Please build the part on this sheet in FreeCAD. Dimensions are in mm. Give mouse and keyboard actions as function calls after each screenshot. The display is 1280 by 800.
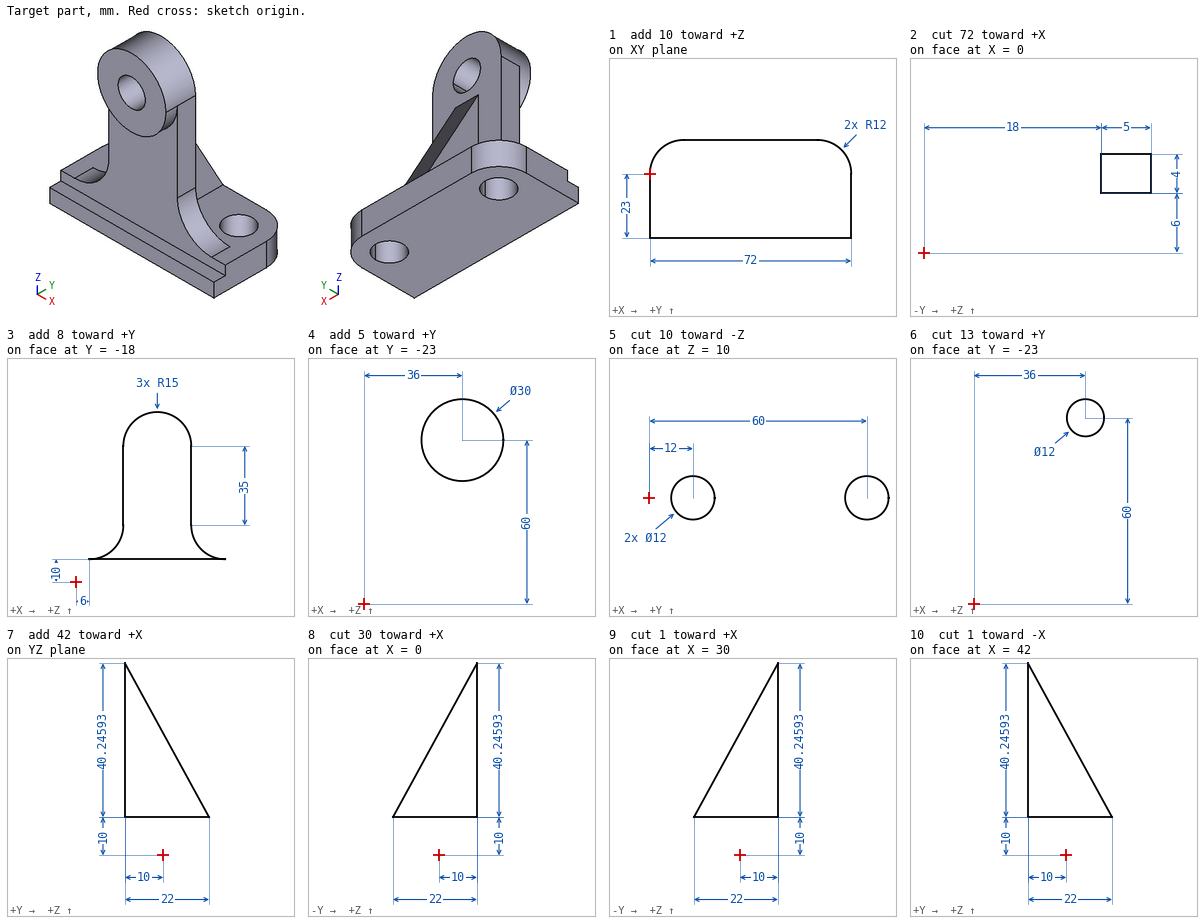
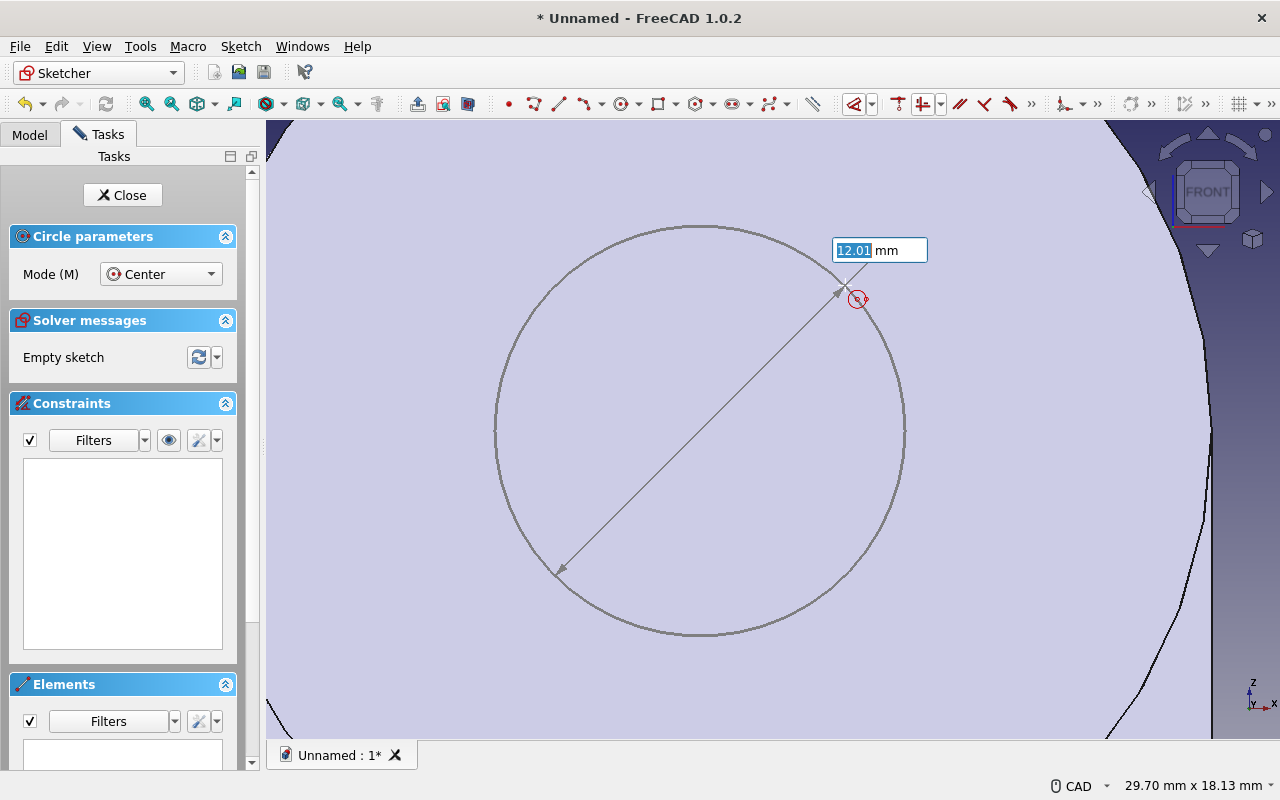
text(12)
key(Return)
key(Escape)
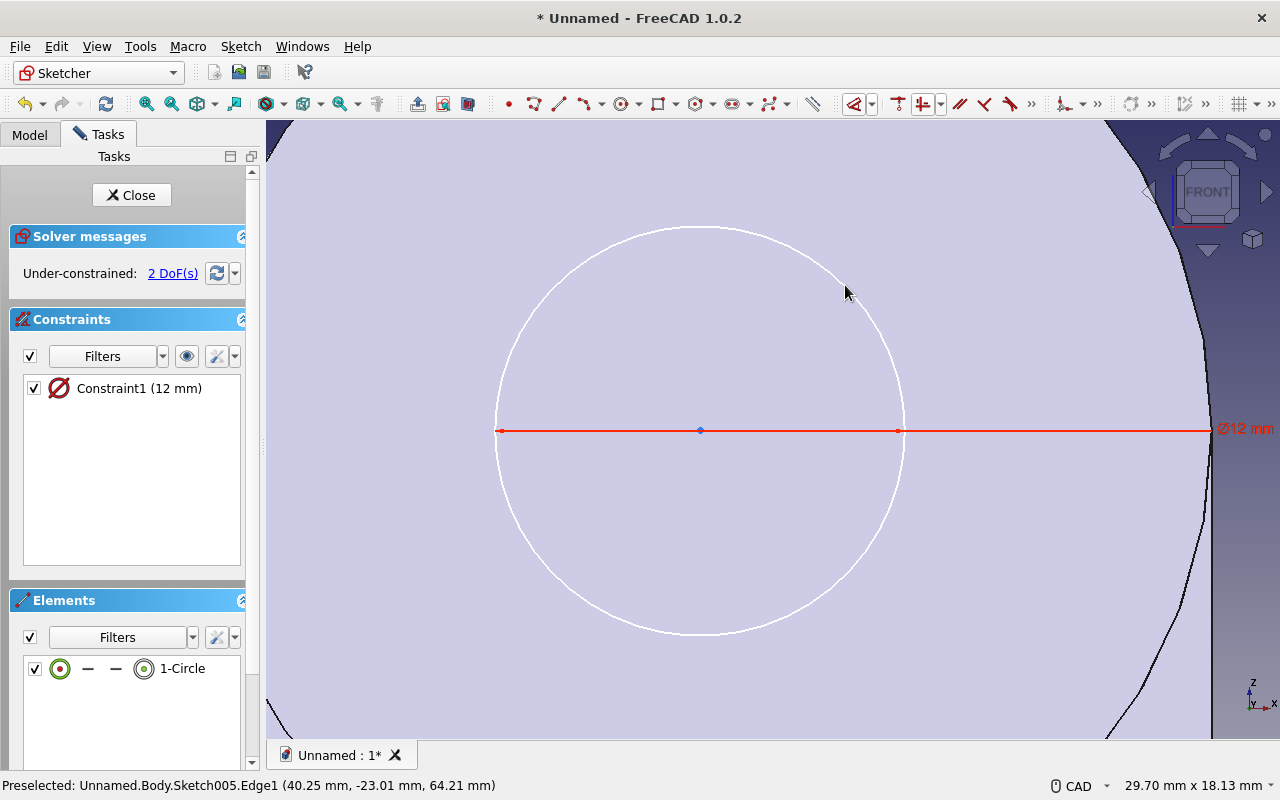
click(700, 431)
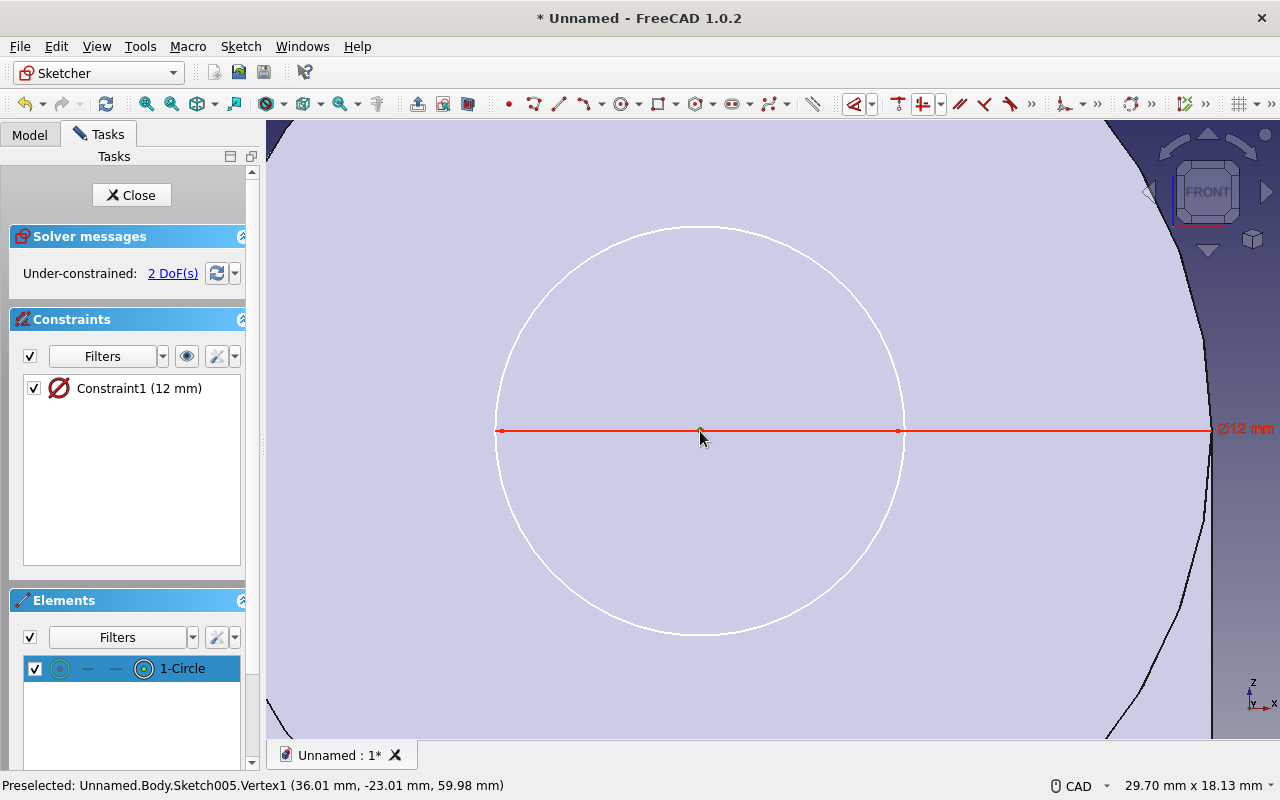
click(872, 104)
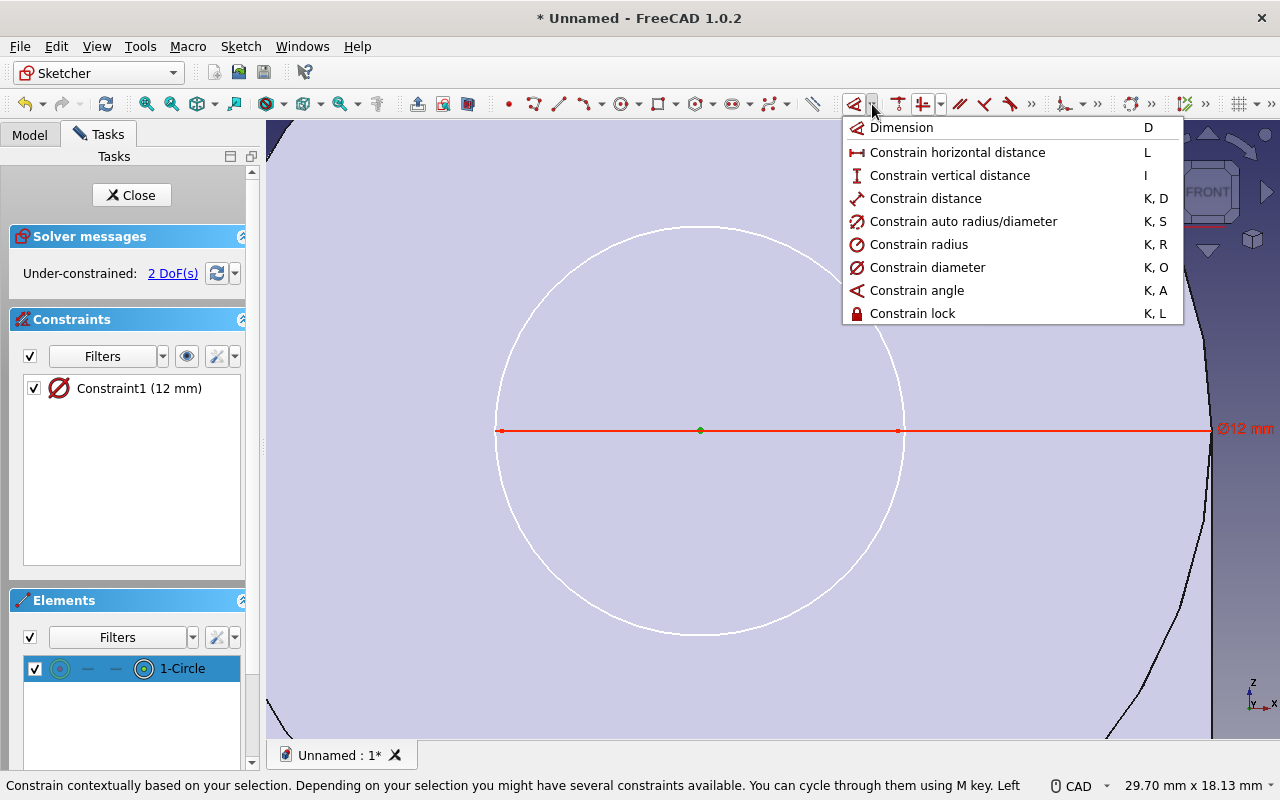
click(1013, 152)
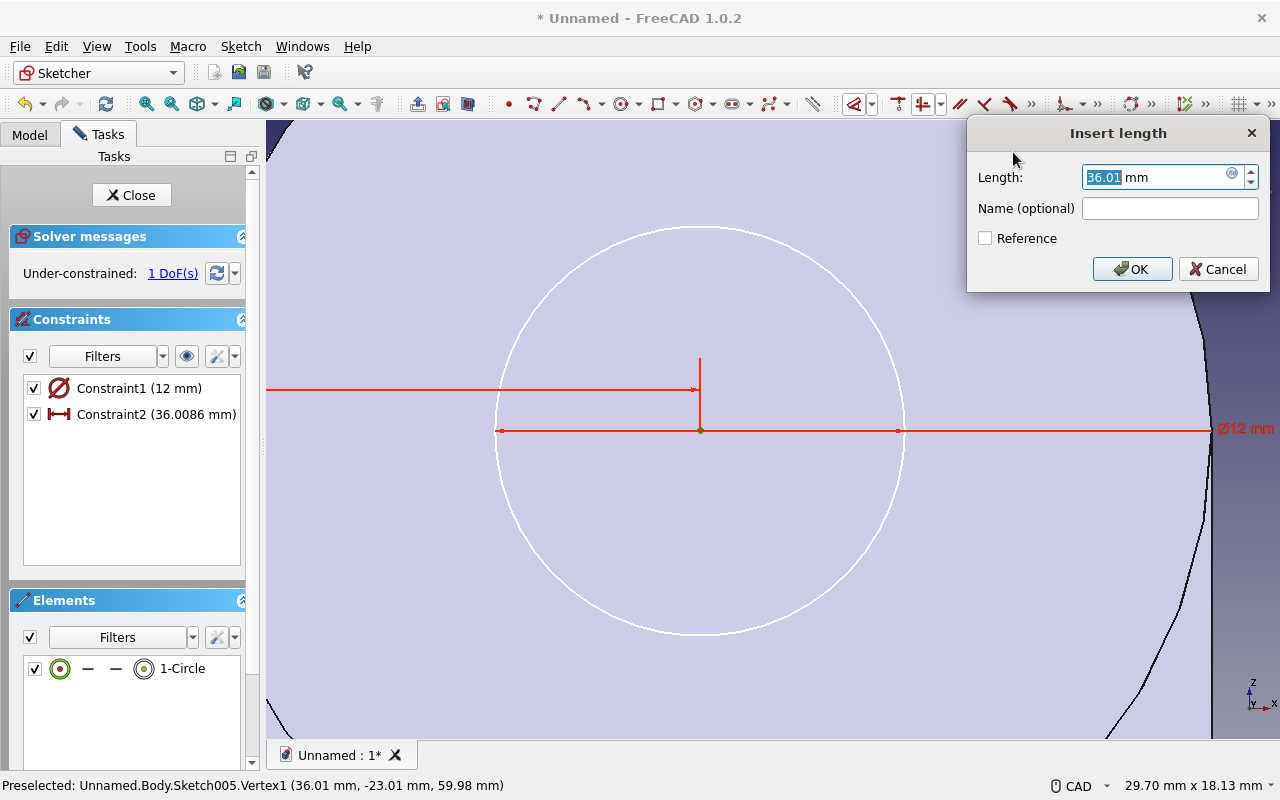
text(36)
key(Return)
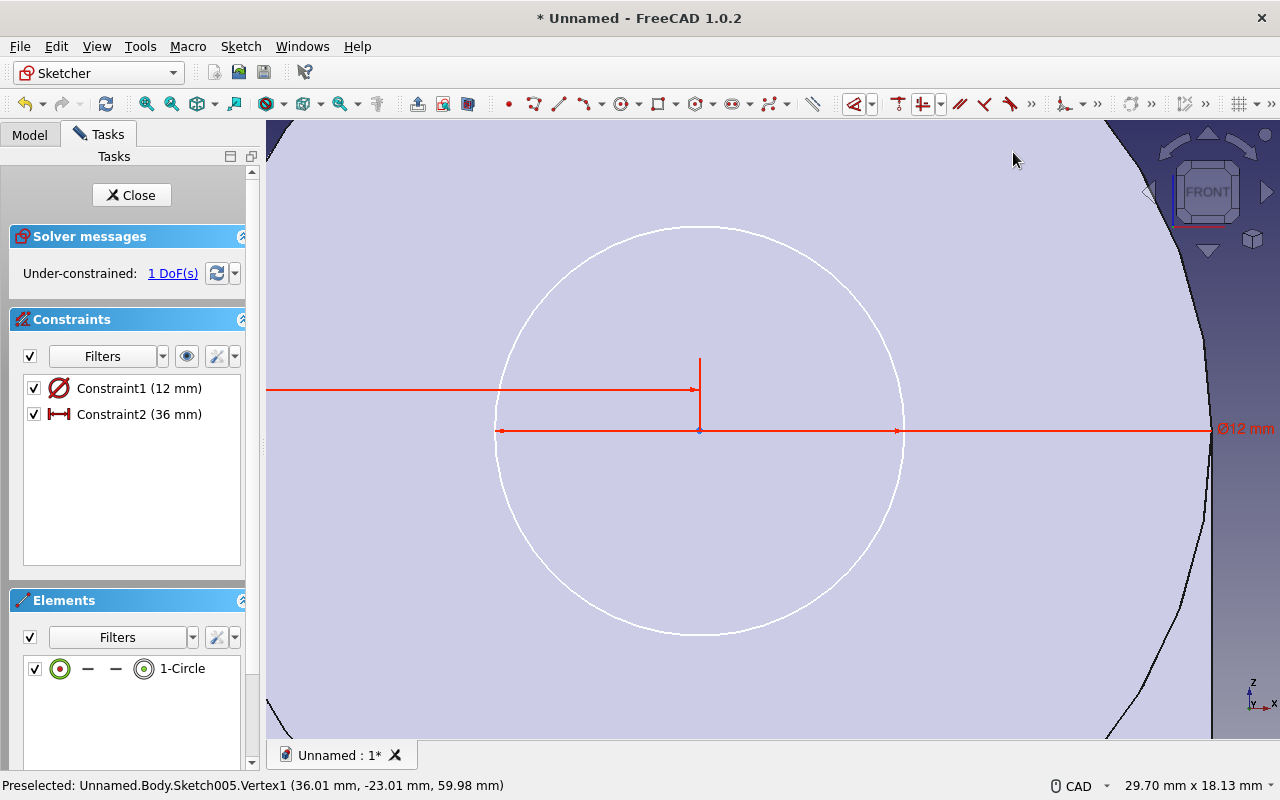
click(700, 431)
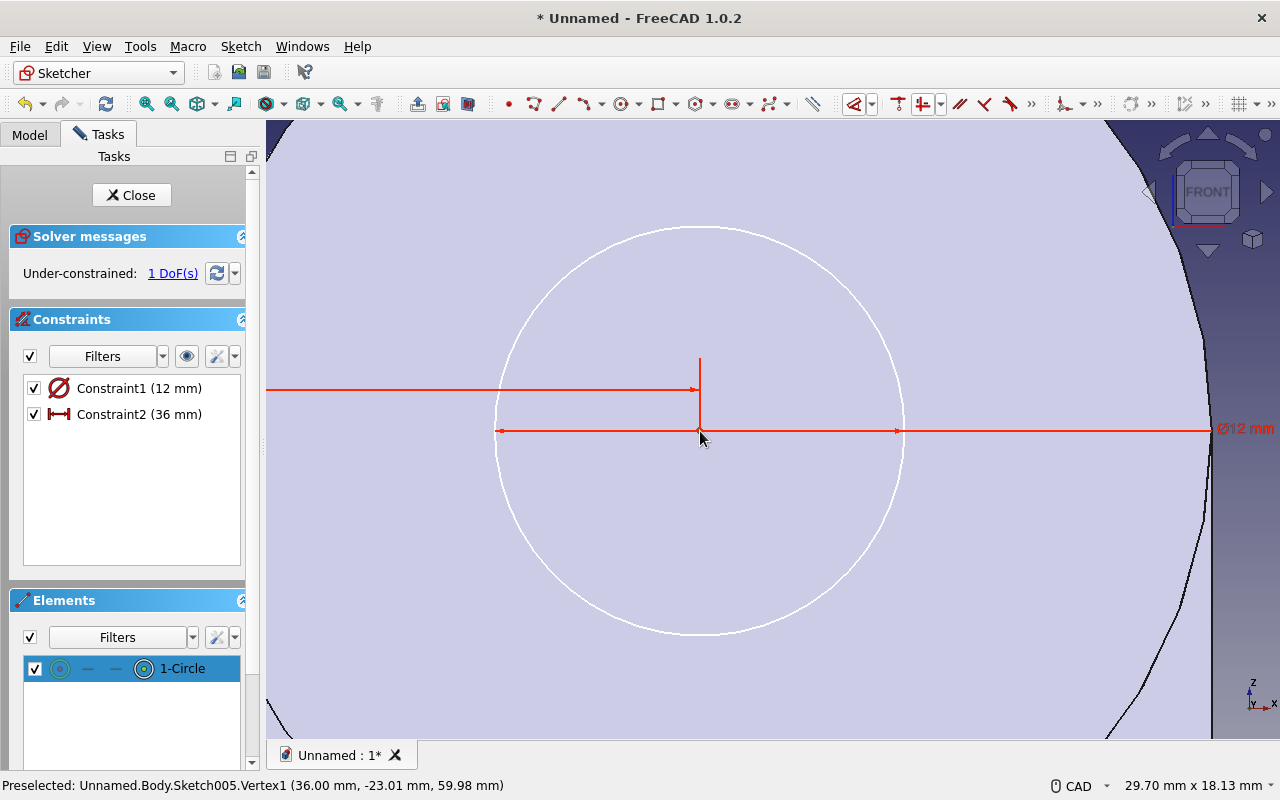
click(872, 104)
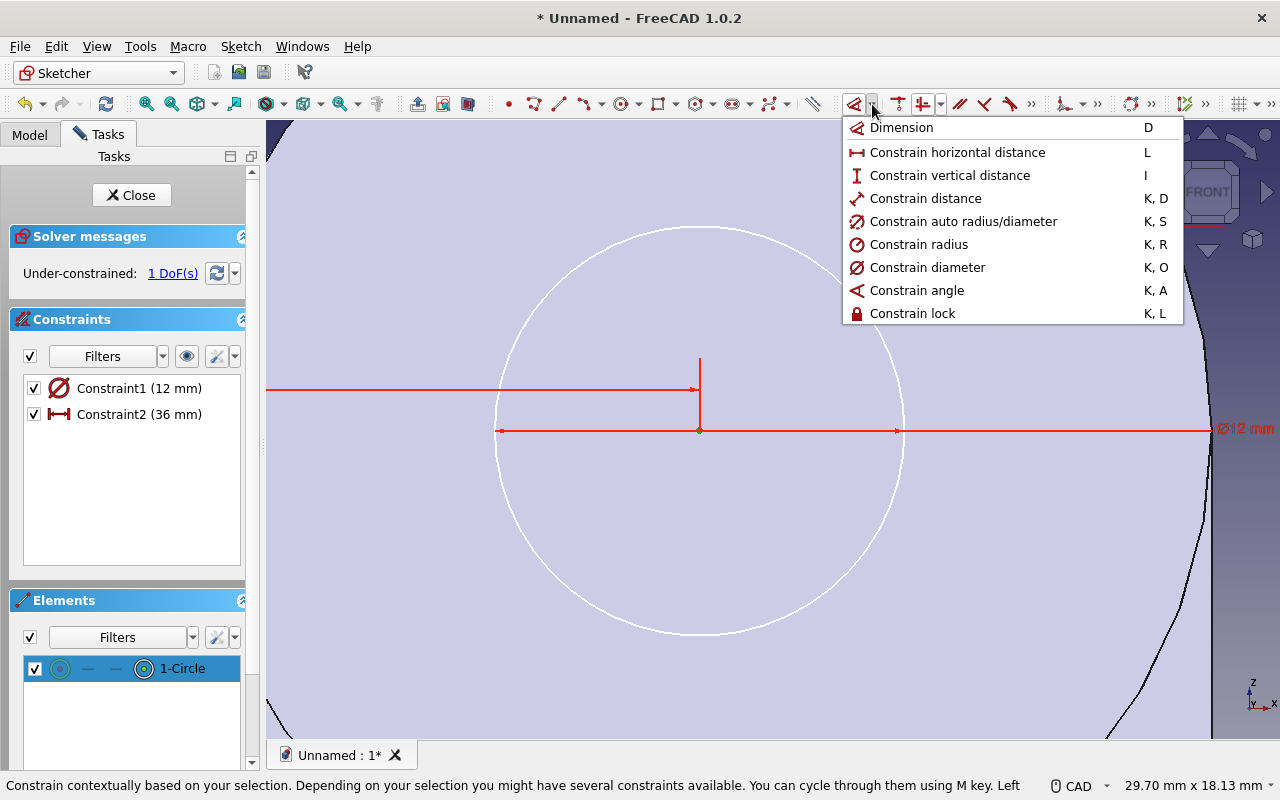
click(1013, 176)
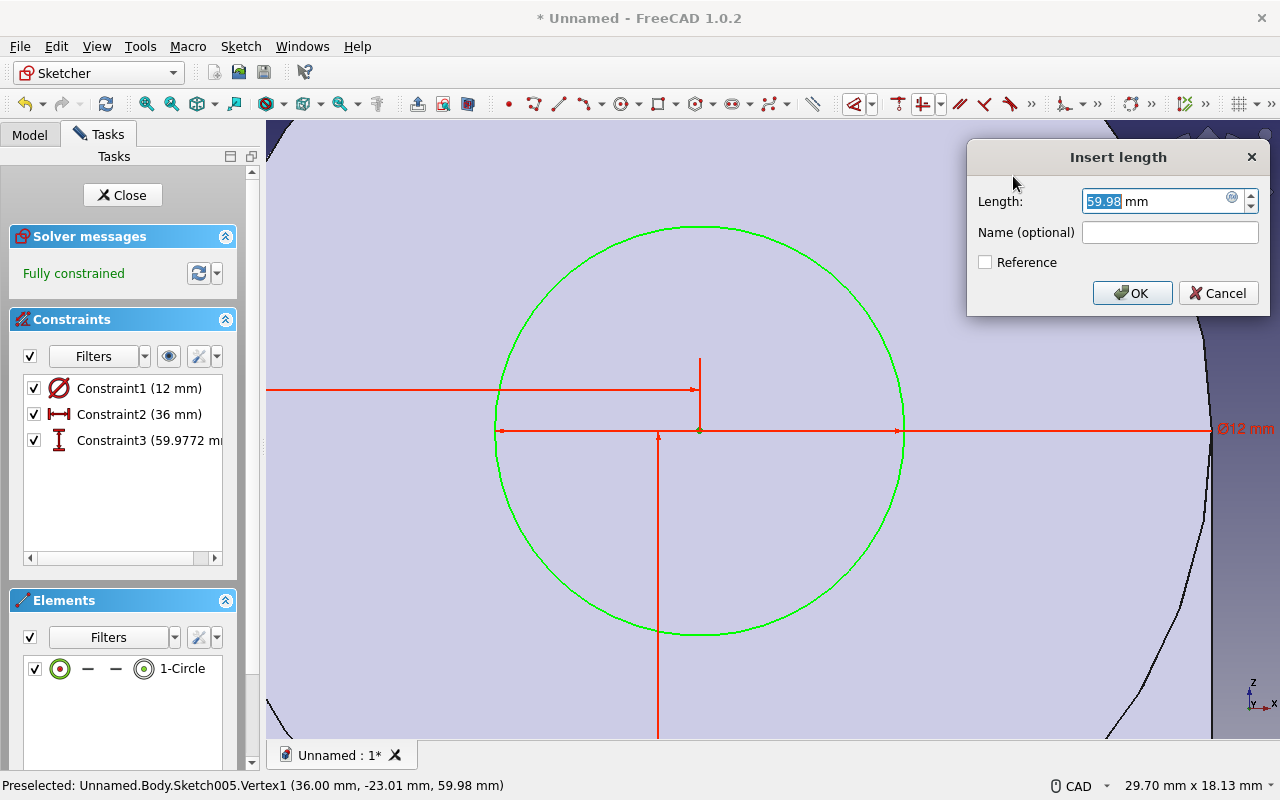
text(60)
key(Return)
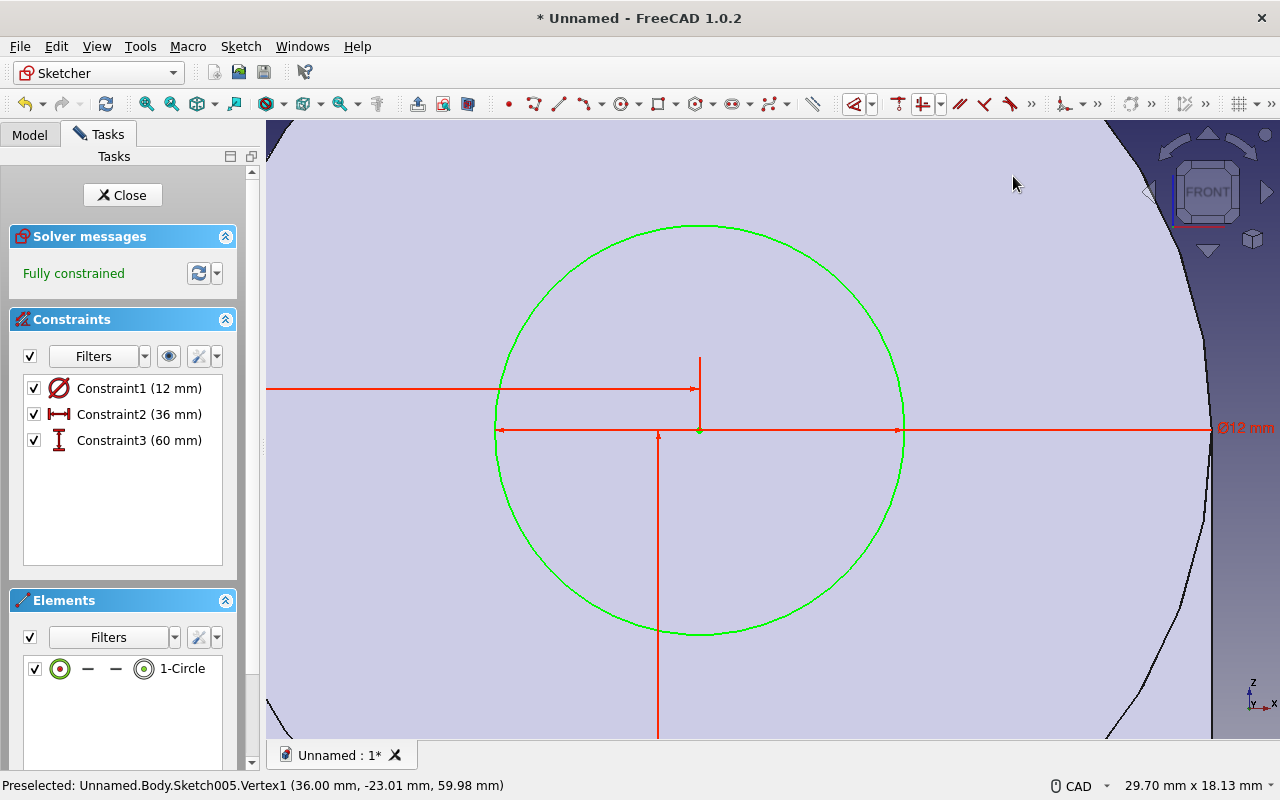
click(123, 195)